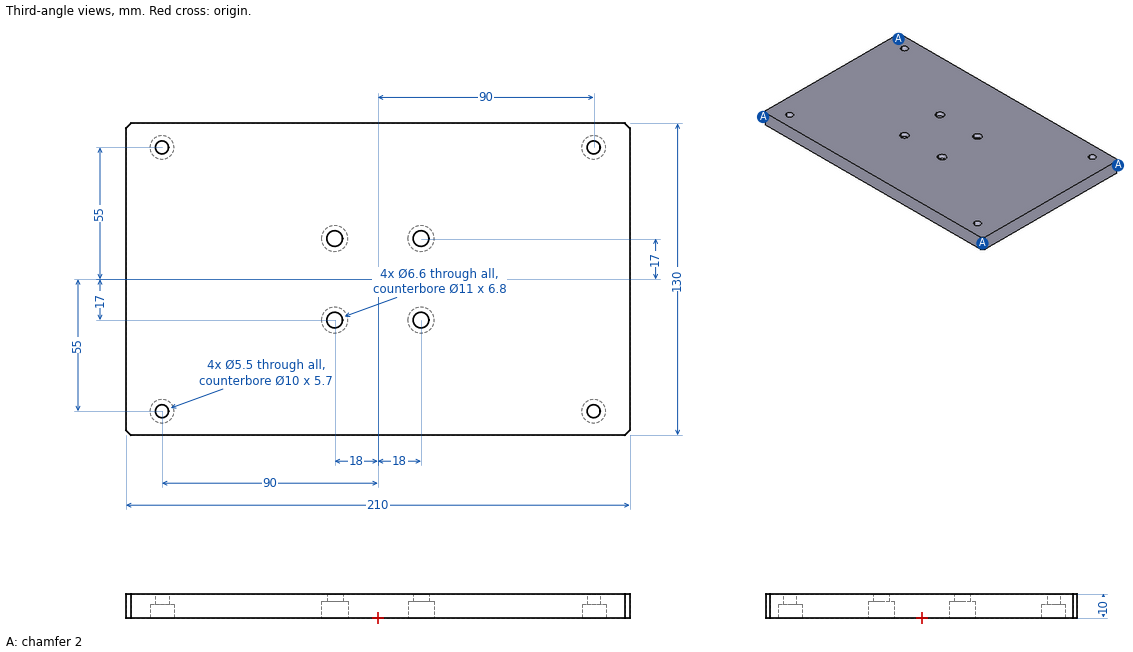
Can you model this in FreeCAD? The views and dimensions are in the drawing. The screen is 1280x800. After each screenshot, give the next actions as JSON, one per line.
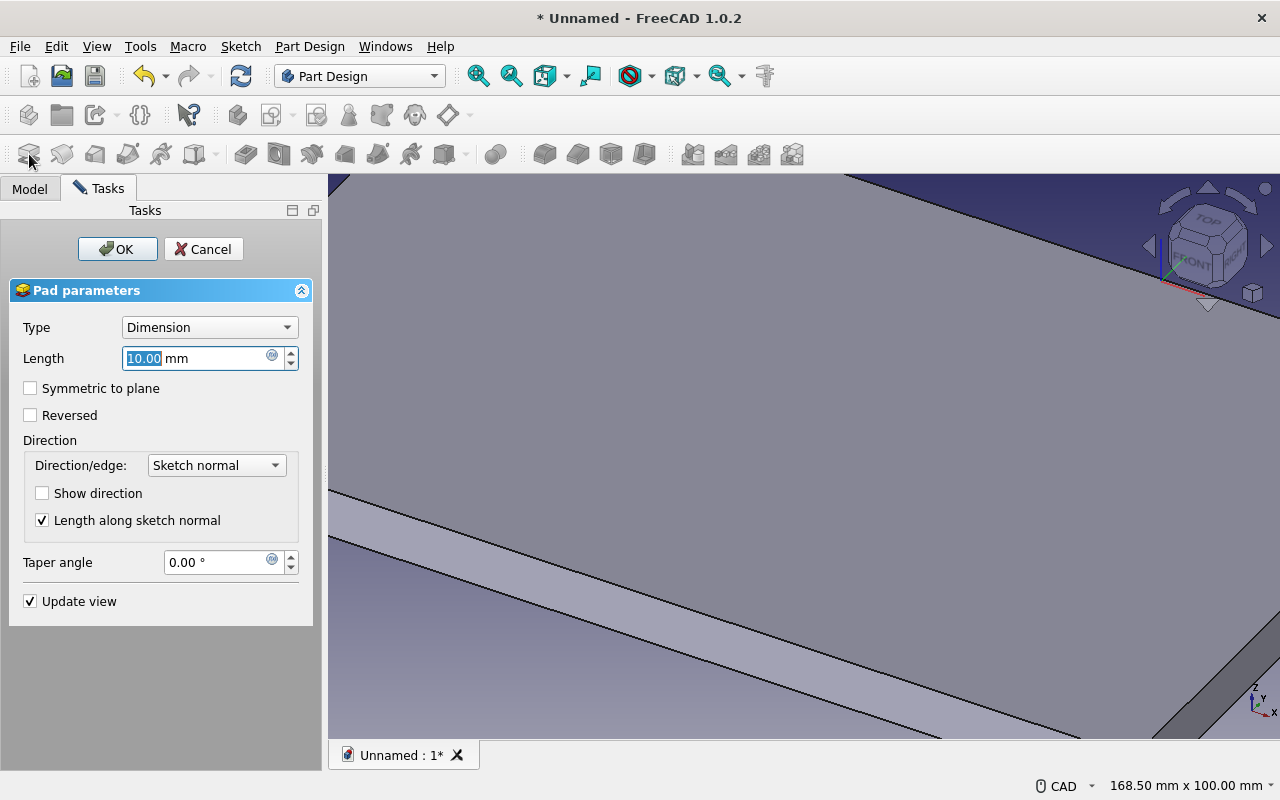
{"action": "type", "text": "10"}
{"action": "key", "text": "Tab"}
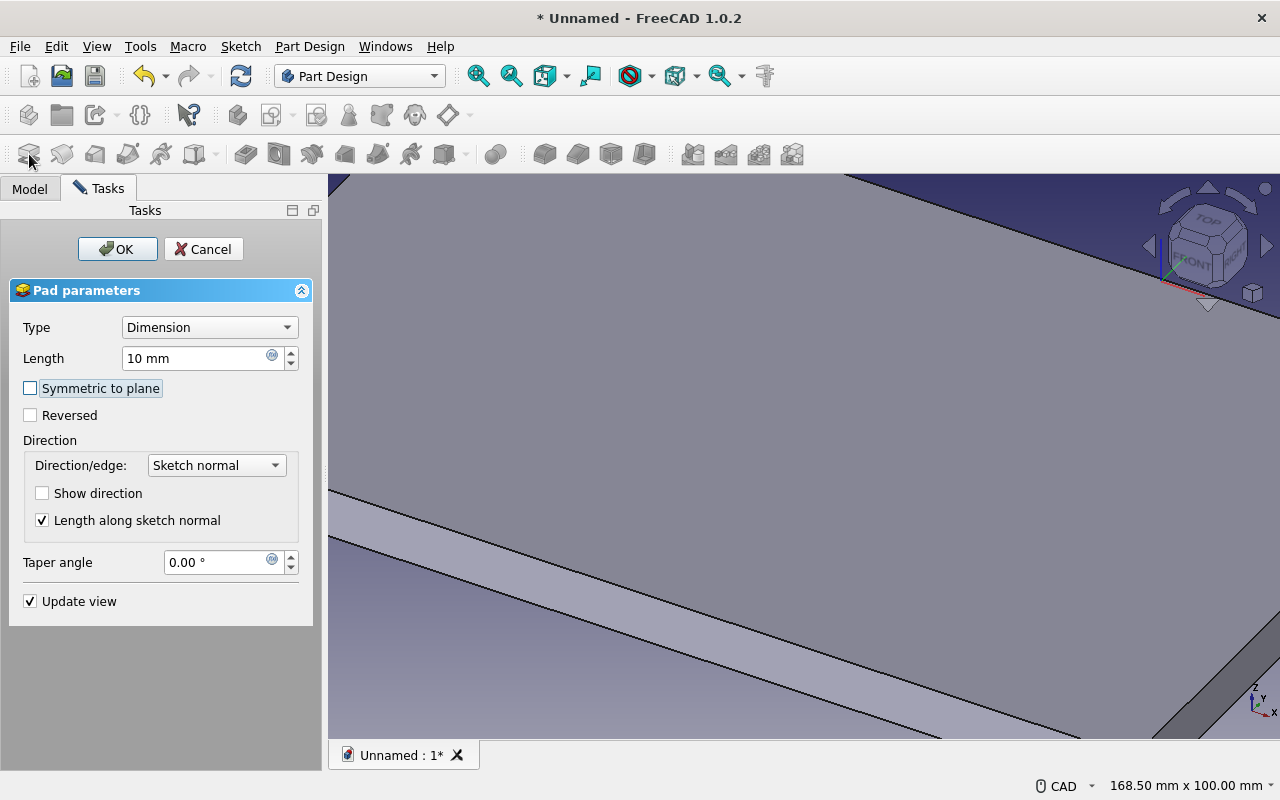
{"action": "left_click", "coordinate": [118, 249]}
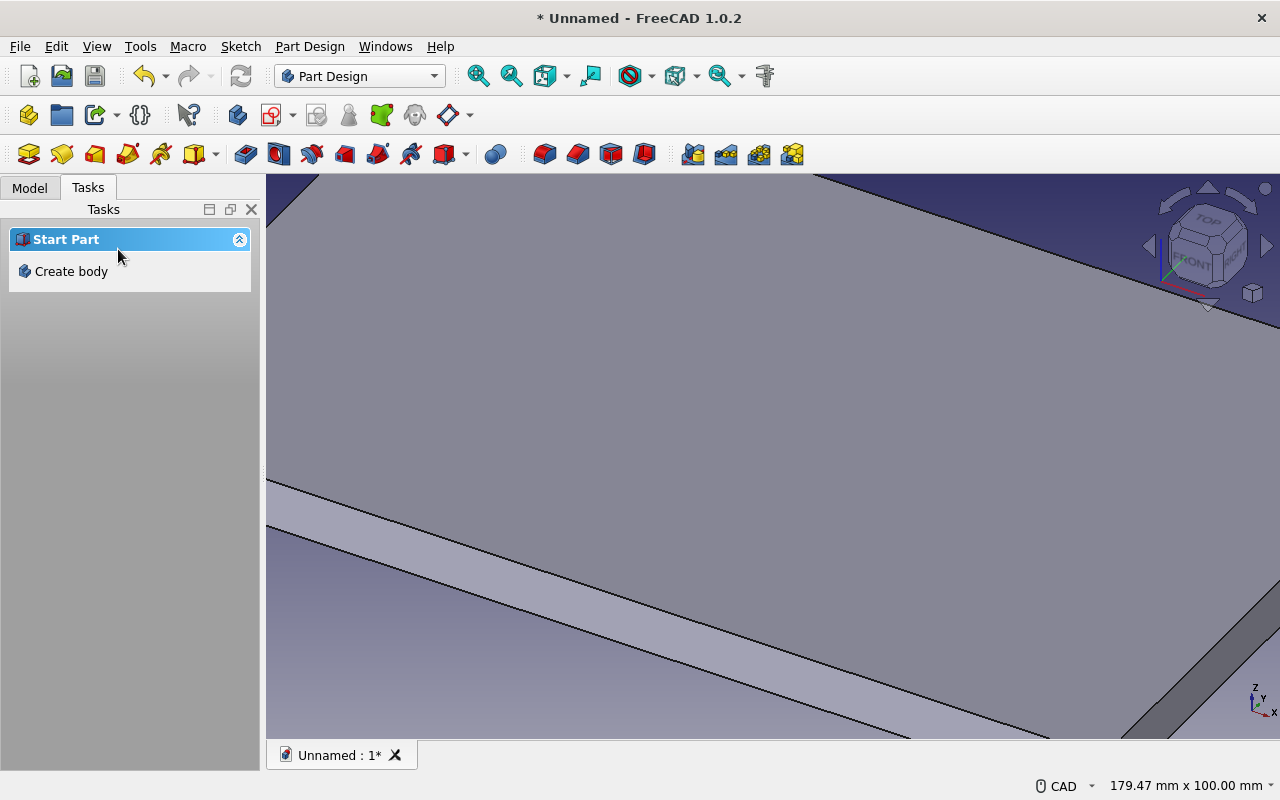
{"action": "key", "text": "v f"}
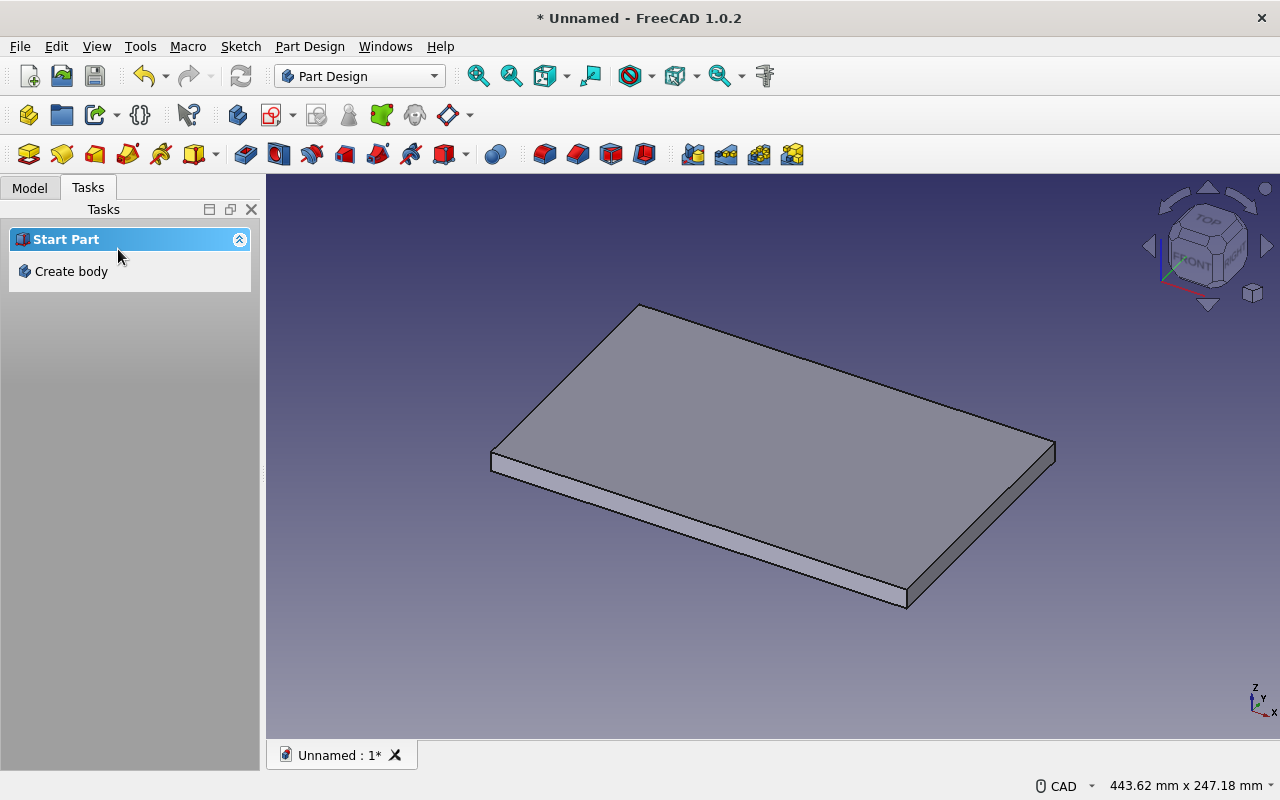
{"action": "left_click", "coordinate": [270, 116]}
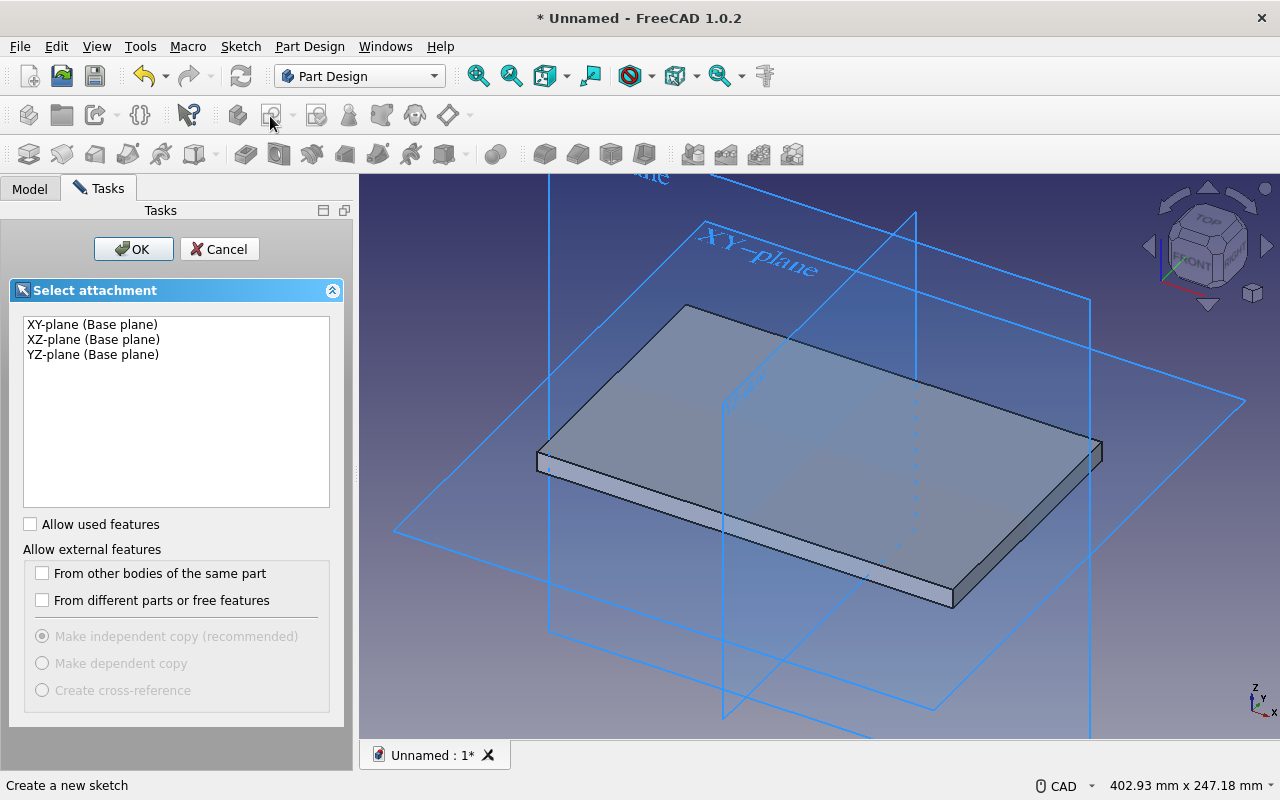
{"action": "left_click", "coordinate": [84, 324]}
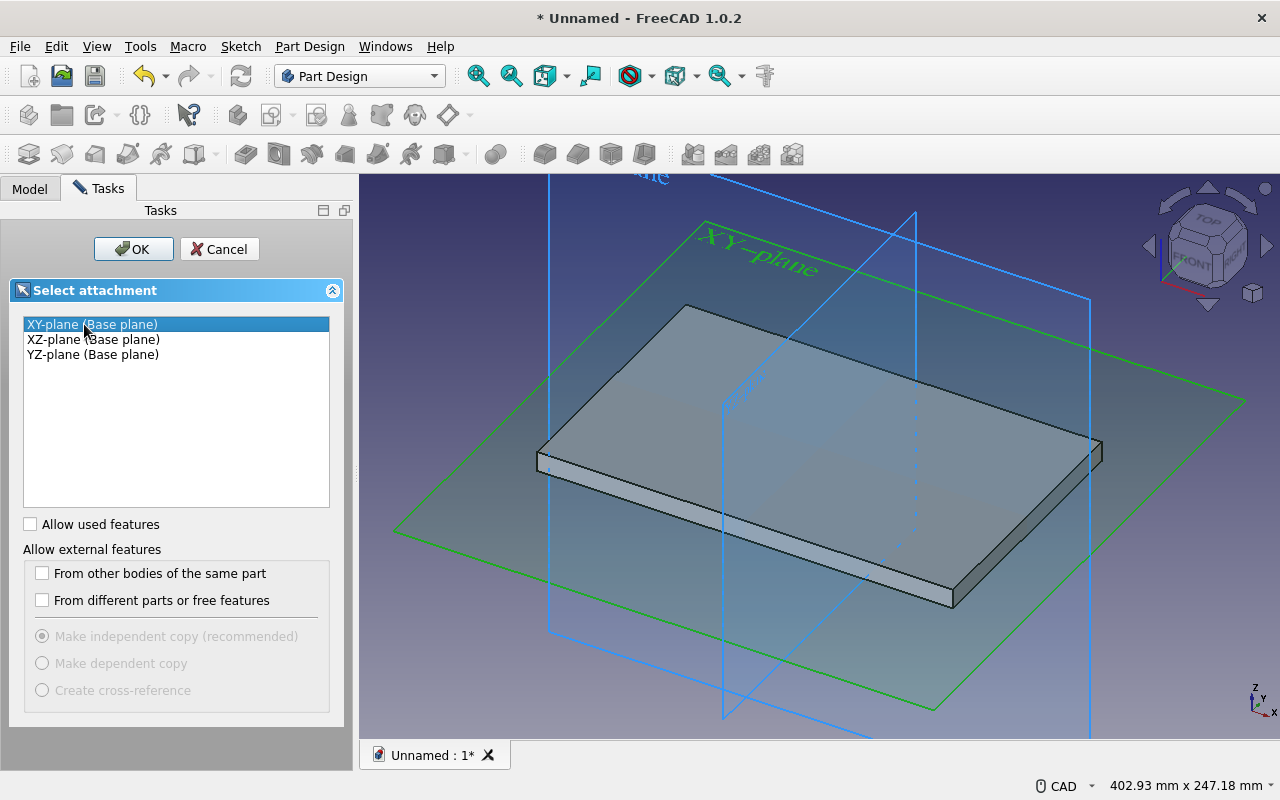
{"action": "left_click", "coordinate": [134, 249]}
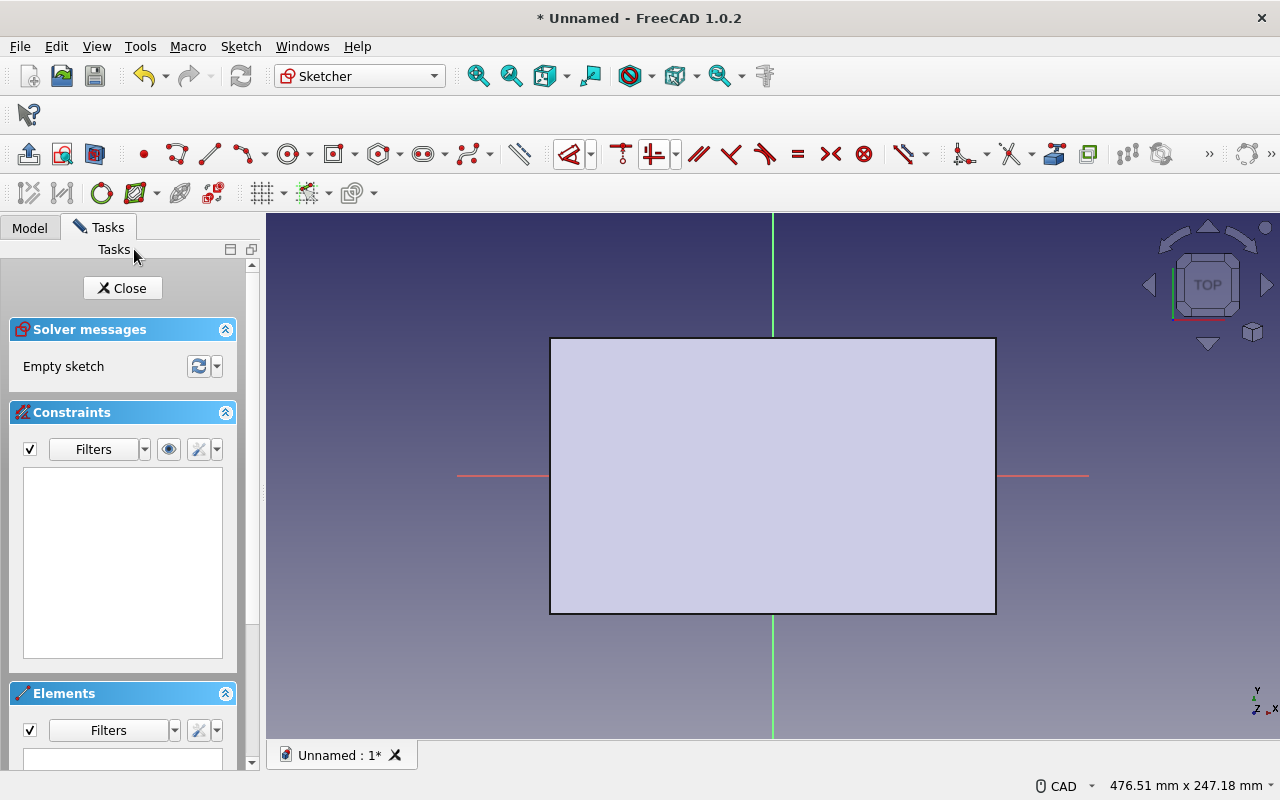
{"action": "key", "text": "q s"}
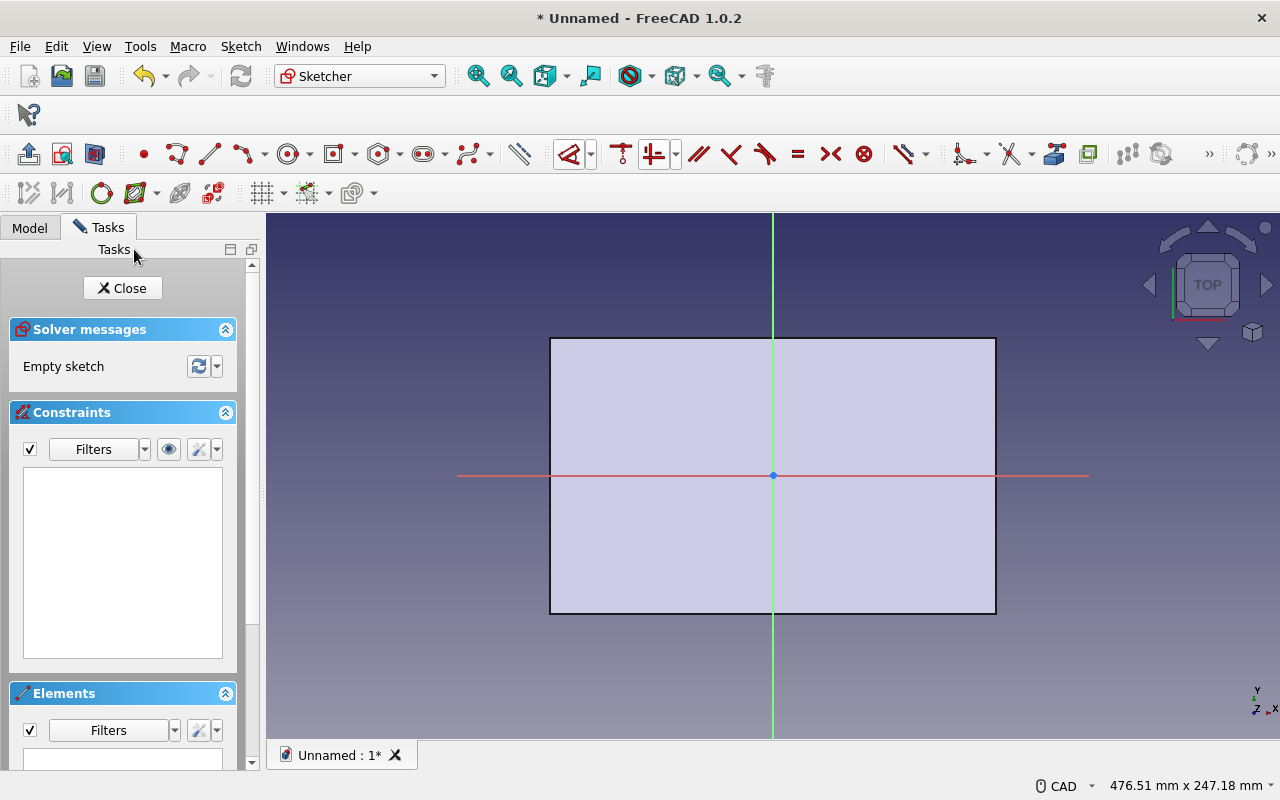
{"action": "scroll", "coordinate": [795, 476], "scroll_direction": "up", "scroll_amount": 7}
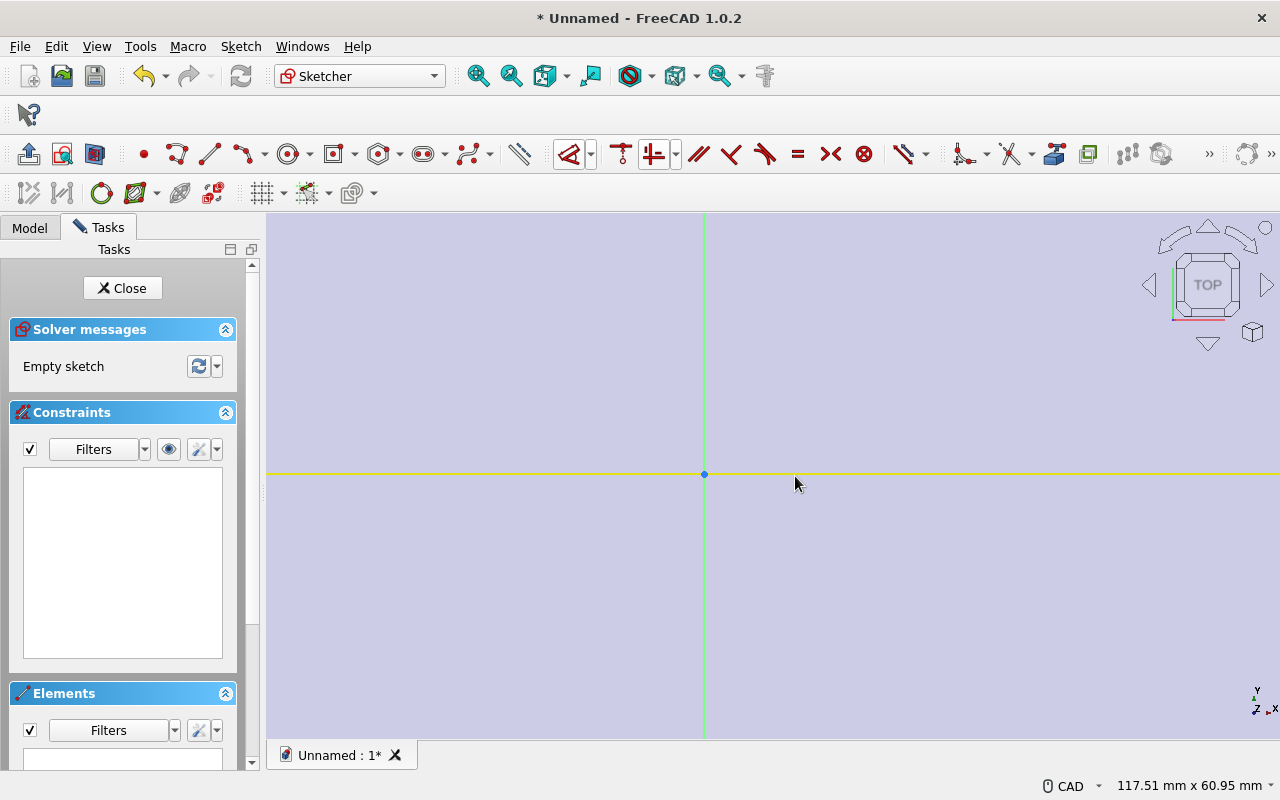
{"action": "key", "text": "g c"}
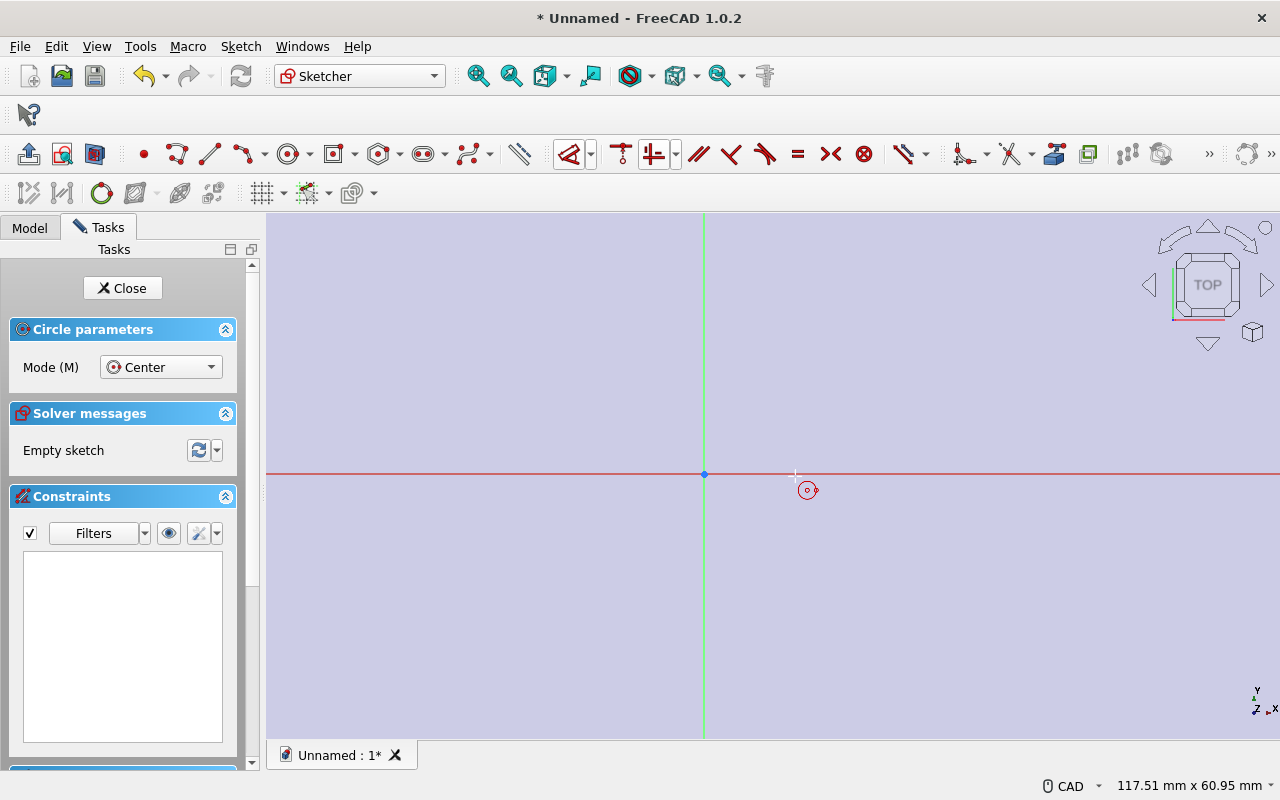
{"action": "left_click", "coordinate": [549, 621]}
{"action": "mouse_move", "coordinate": [569, 601]}